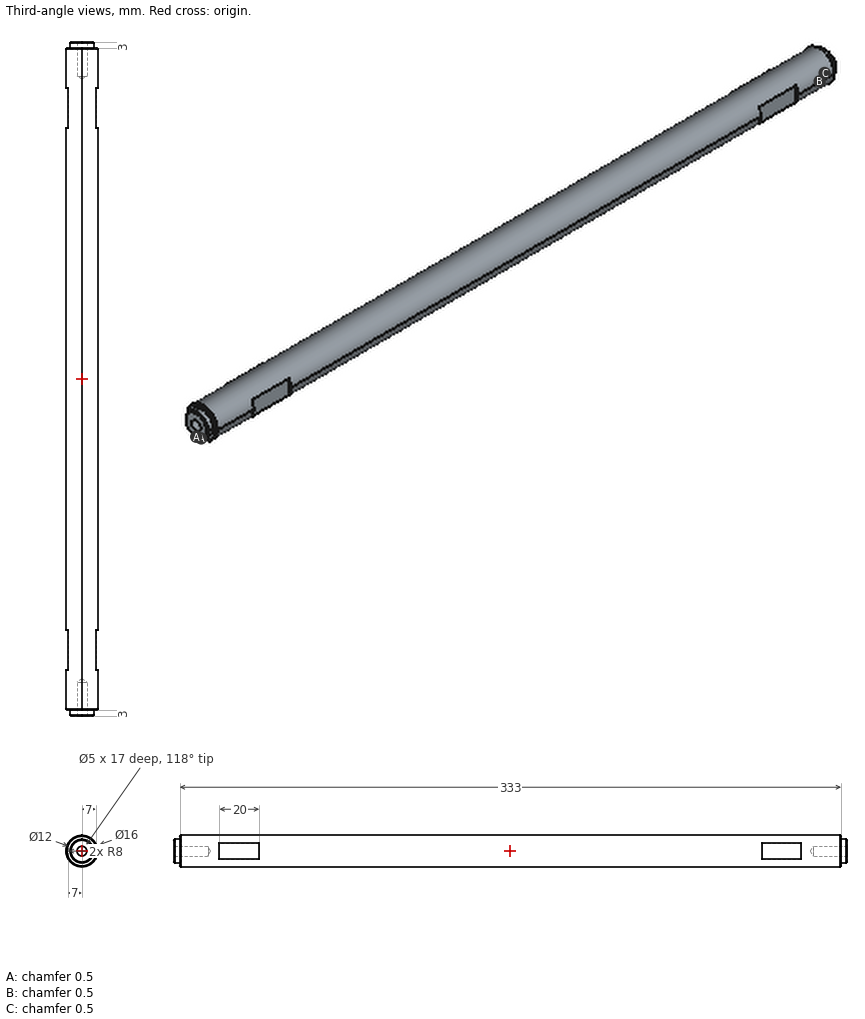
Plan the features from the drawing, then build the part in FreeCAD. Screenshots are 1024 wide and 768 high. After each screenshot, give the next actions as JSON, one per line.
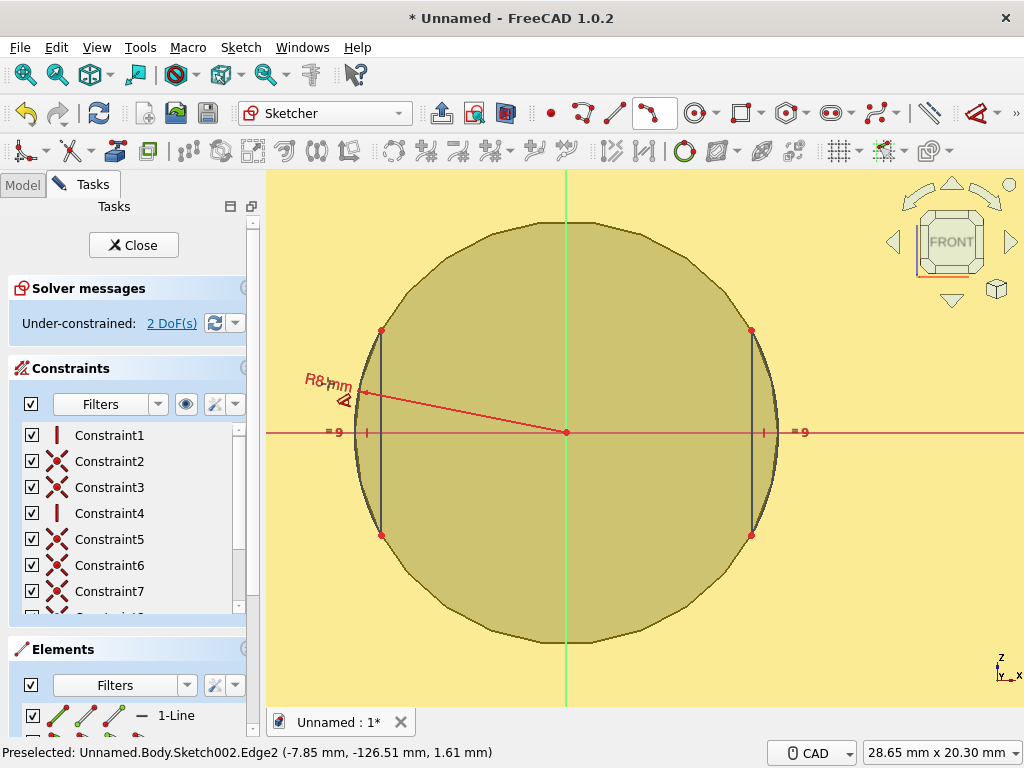
{"action": "left_click", "coordinate": [381, 535]}
{"action": "left_click", "coordinate": [474, 569]}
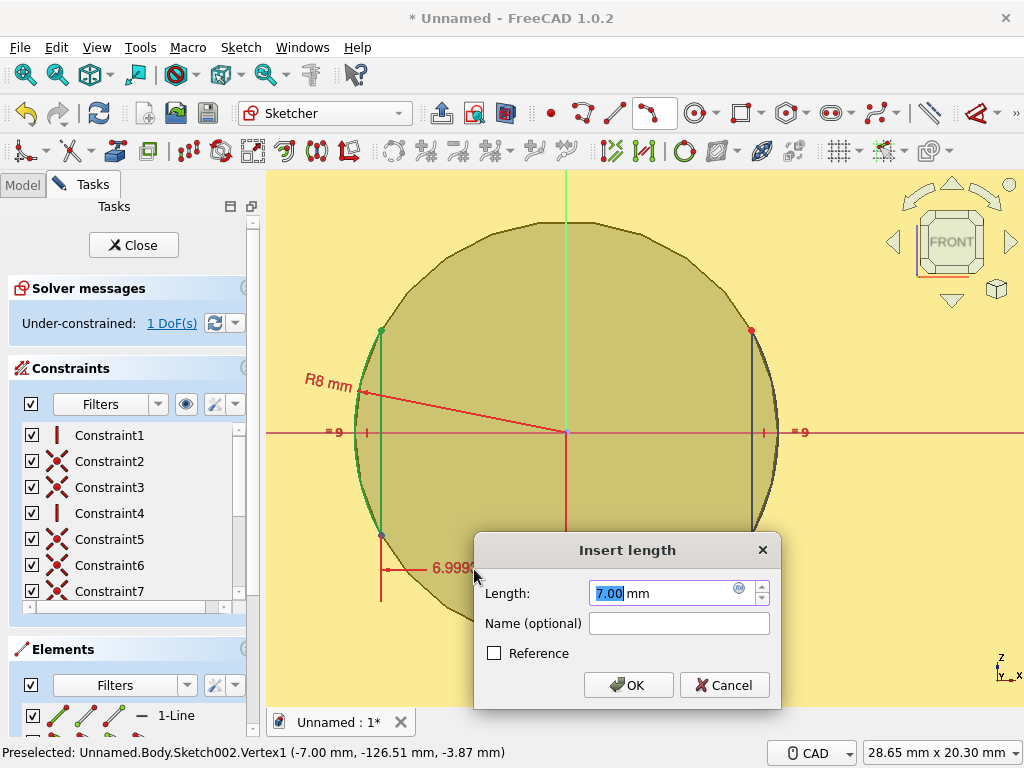
{"action": "type", "text": "7"}
{"action": "key", "text": "Return"}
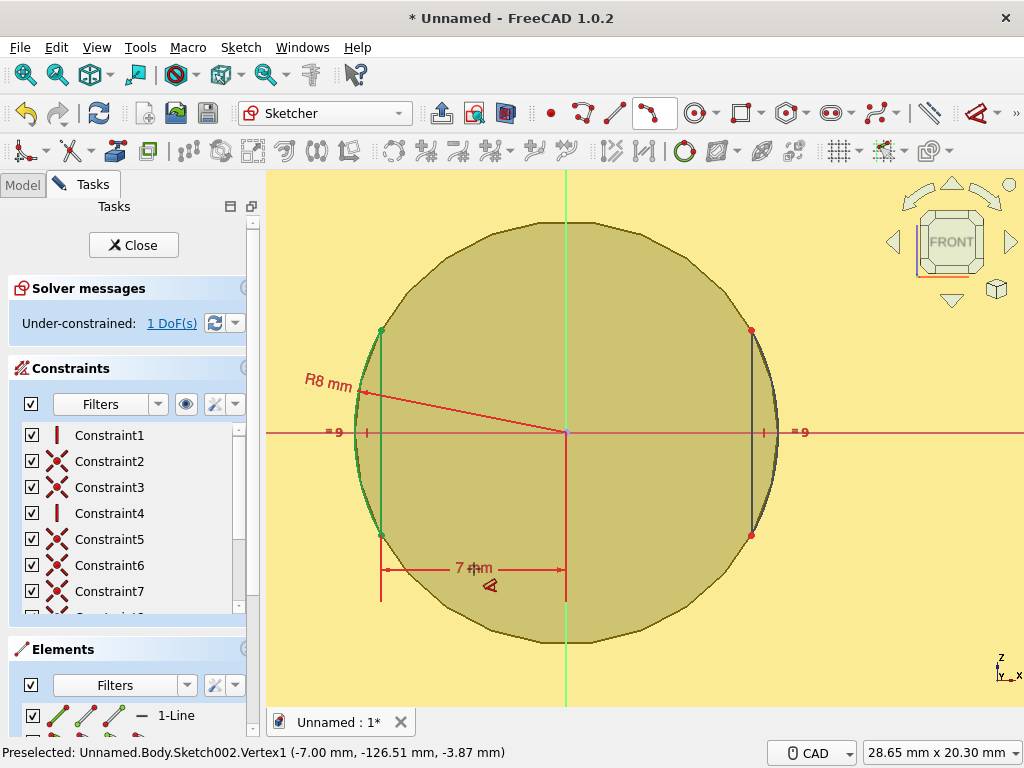
{"action": "left_click", "coordinate": [752, 330]}
{"action": "left_click", "coordinate": [659, 296]}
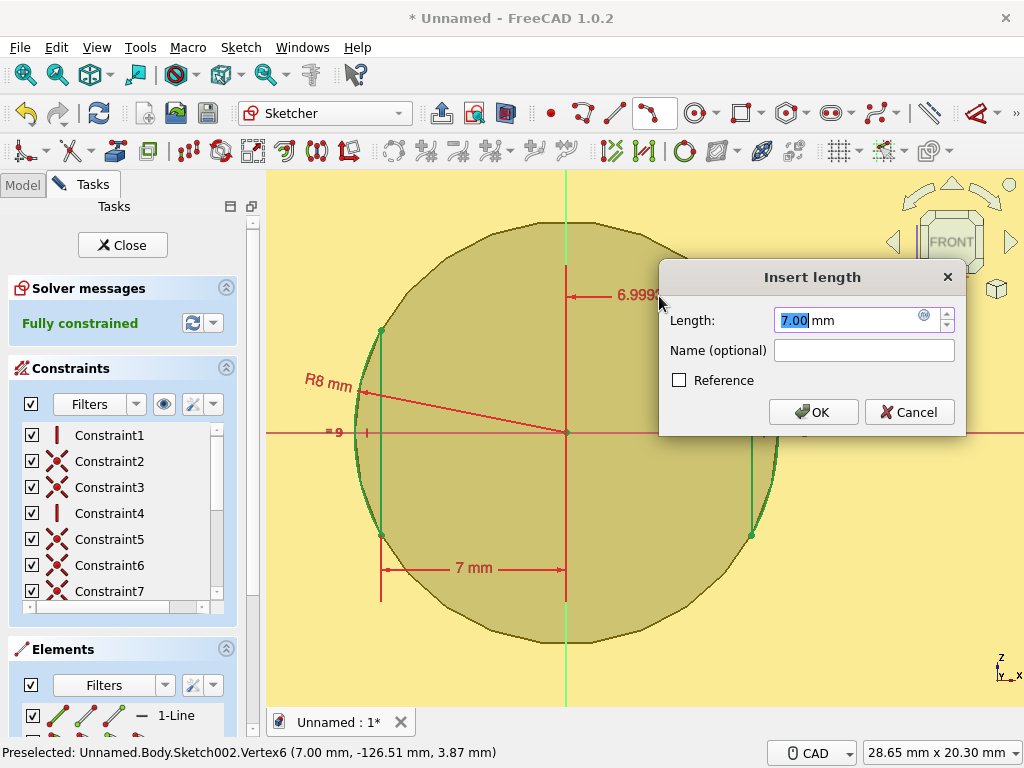
{"action": "type", "text": "7"}
{"action": "key", "text": "Return"}
{"action": "key", "text": "Escape"}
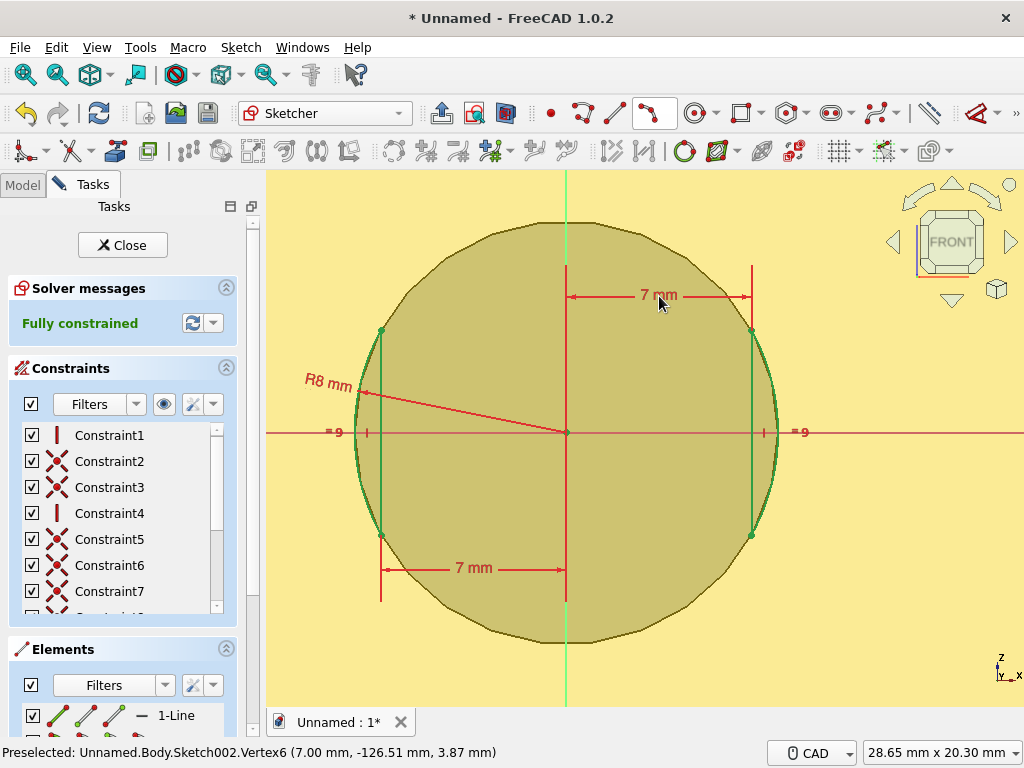
{"action": "left_click", "coordinate": [123, 245]}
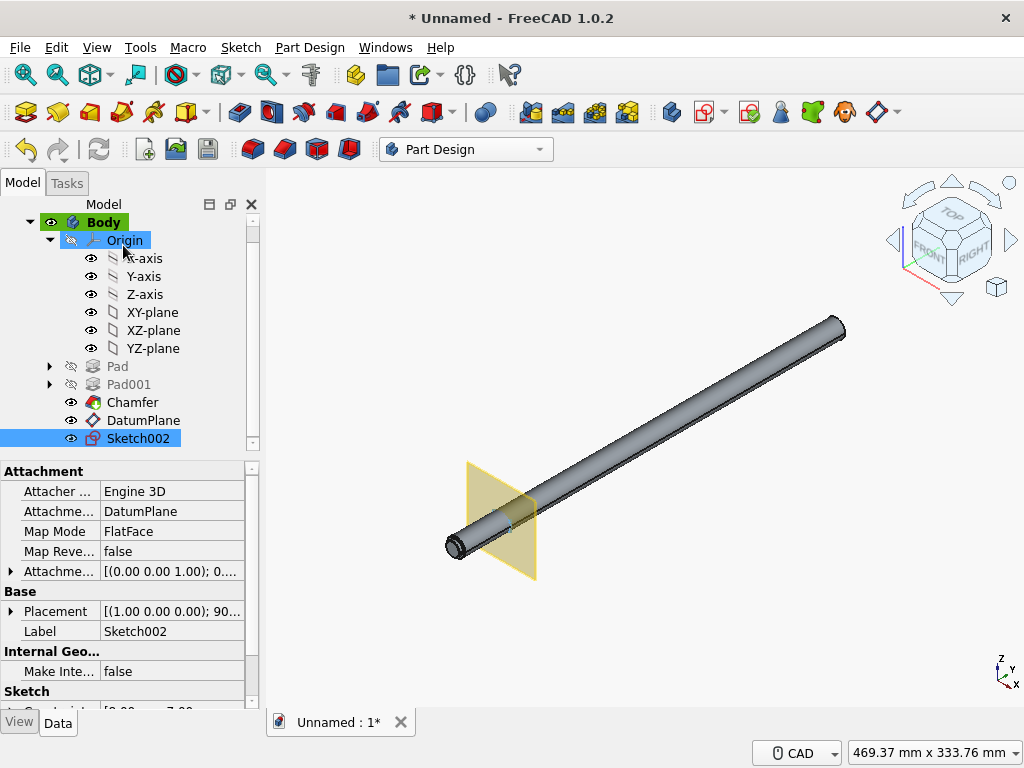
{"action": "left_click", "coordinate": [240, 112]}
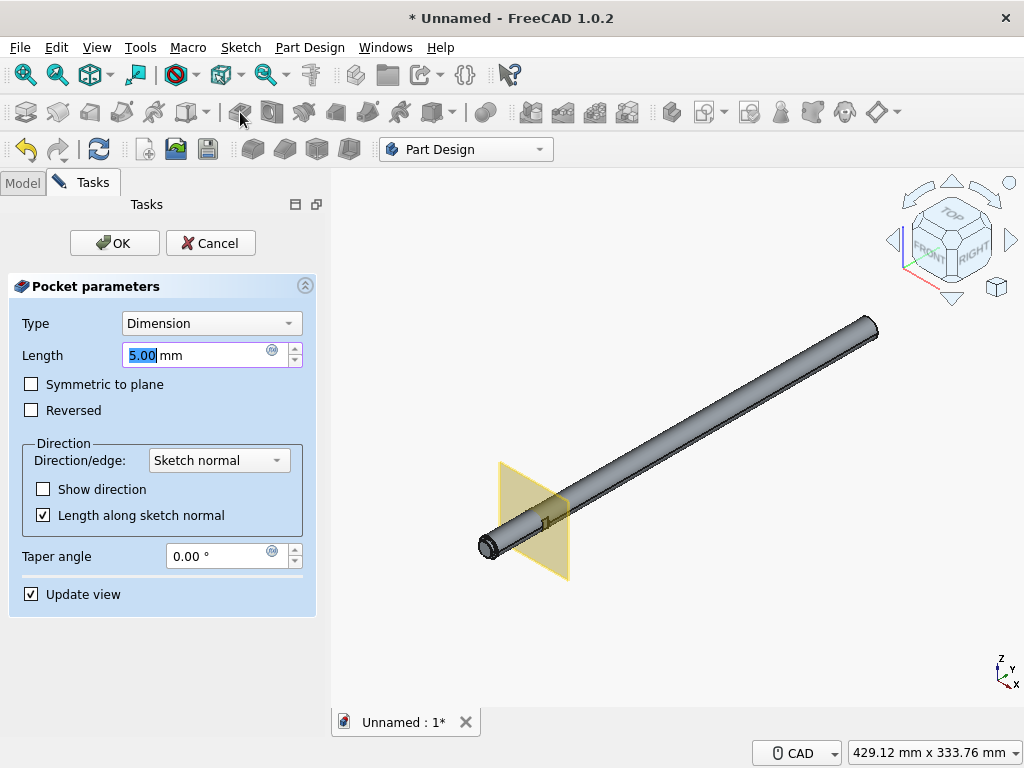
{"action": "type", "text": "20"}
{"action": "key", "text": "Tab"}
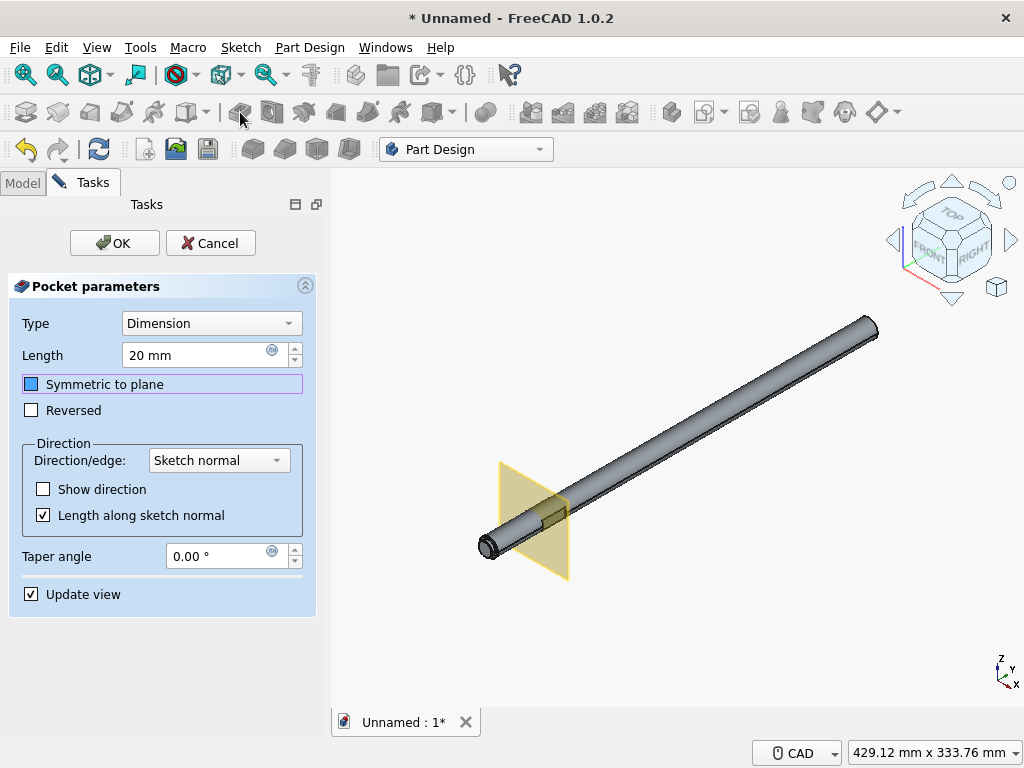
{"action": "left_click", "coordinate": [30, 410]}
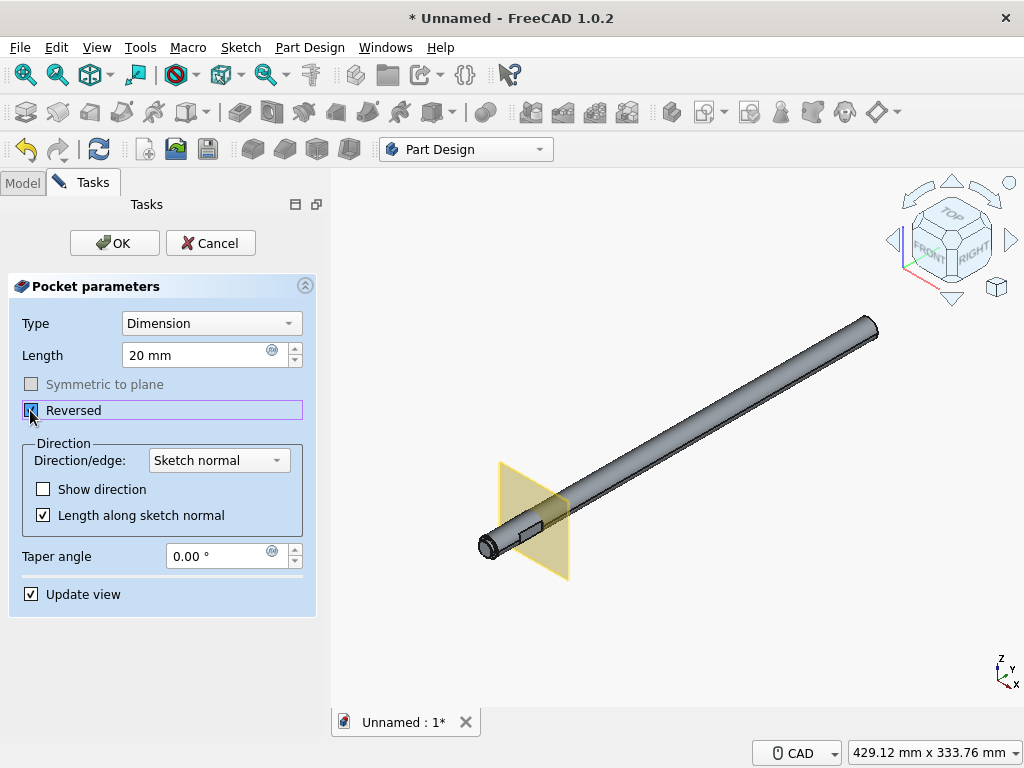
{"action": "left_click", "coordinate": [115, 243]}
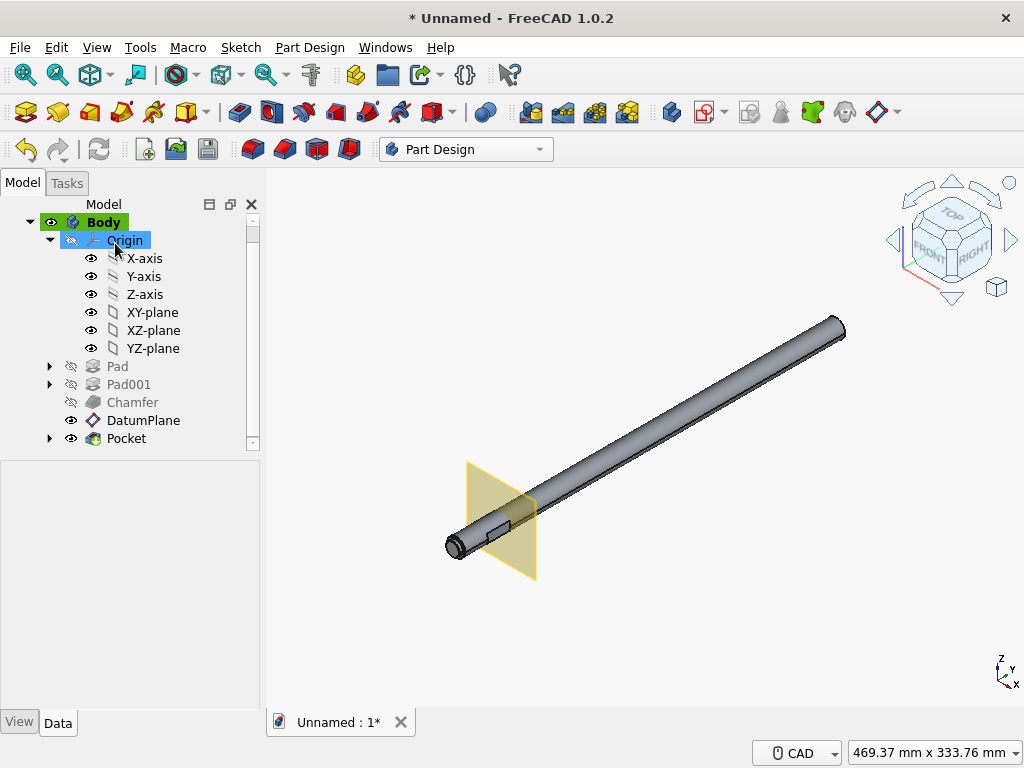
{"action": "left_click", "coordinate": [116, 420]}
{"action": "key", "text": "space"}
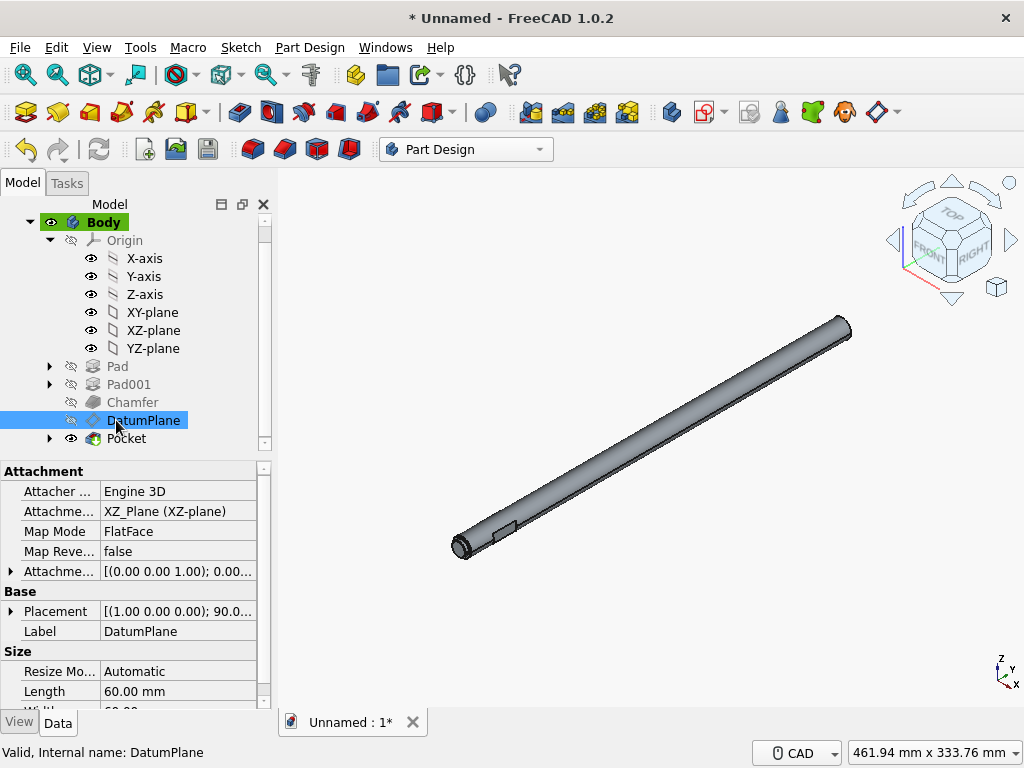
{"action": "key", "text": "1"}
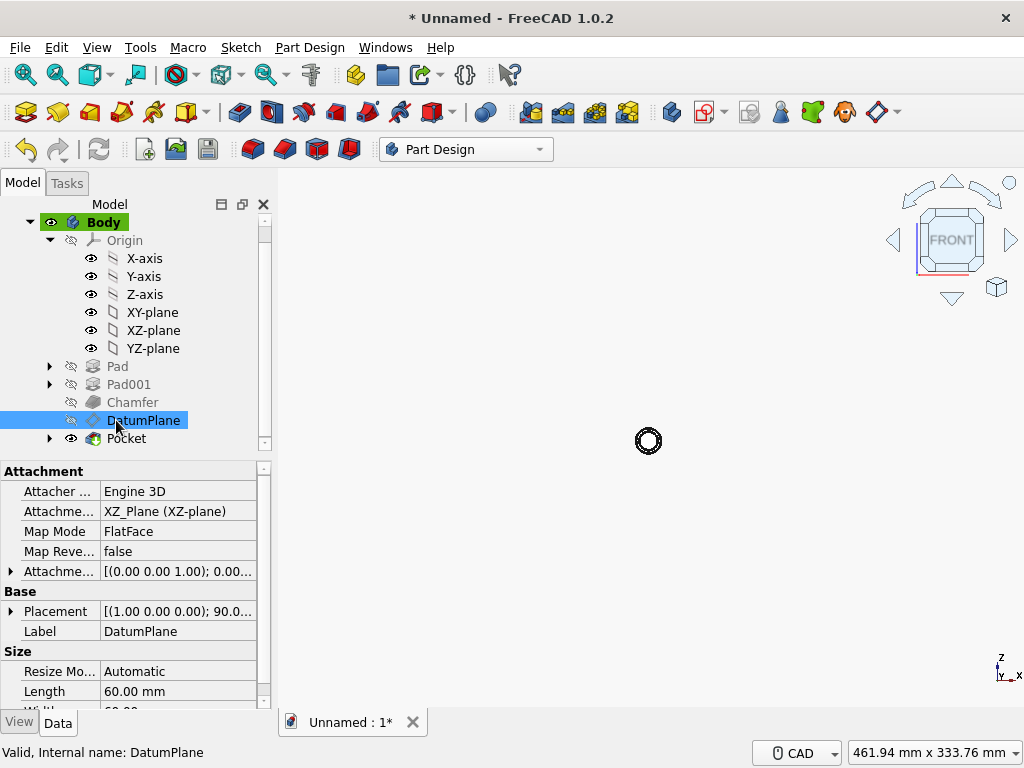
{"action": "key", "text": "v f"}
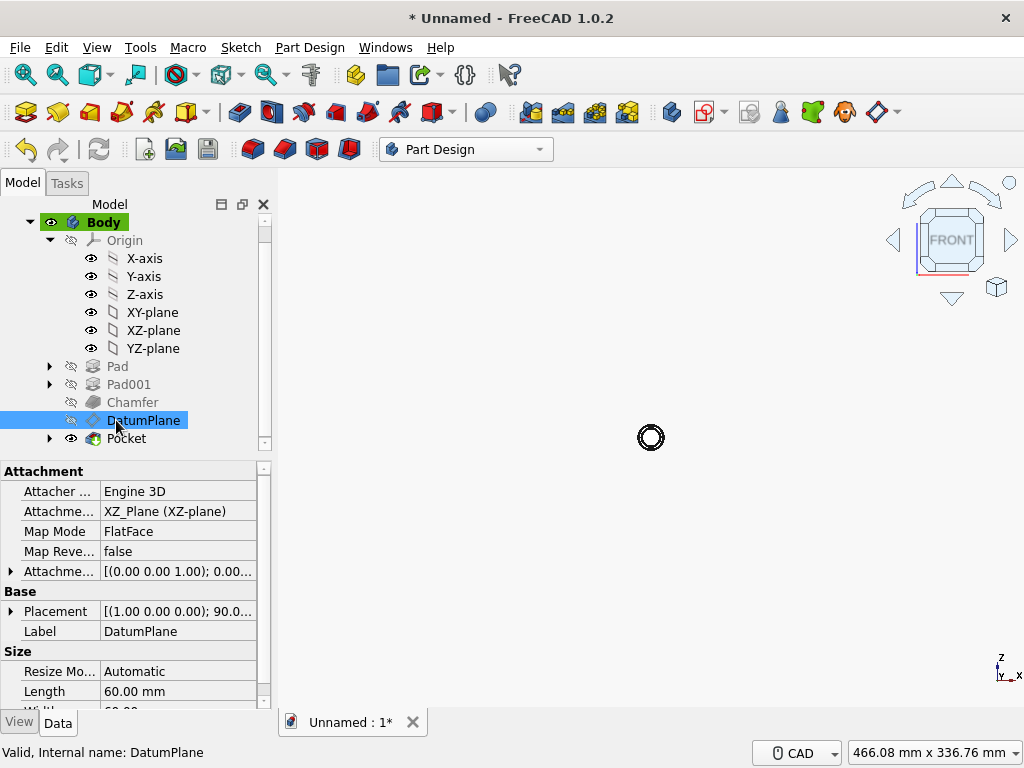
{"action": "key", "text": "0"}